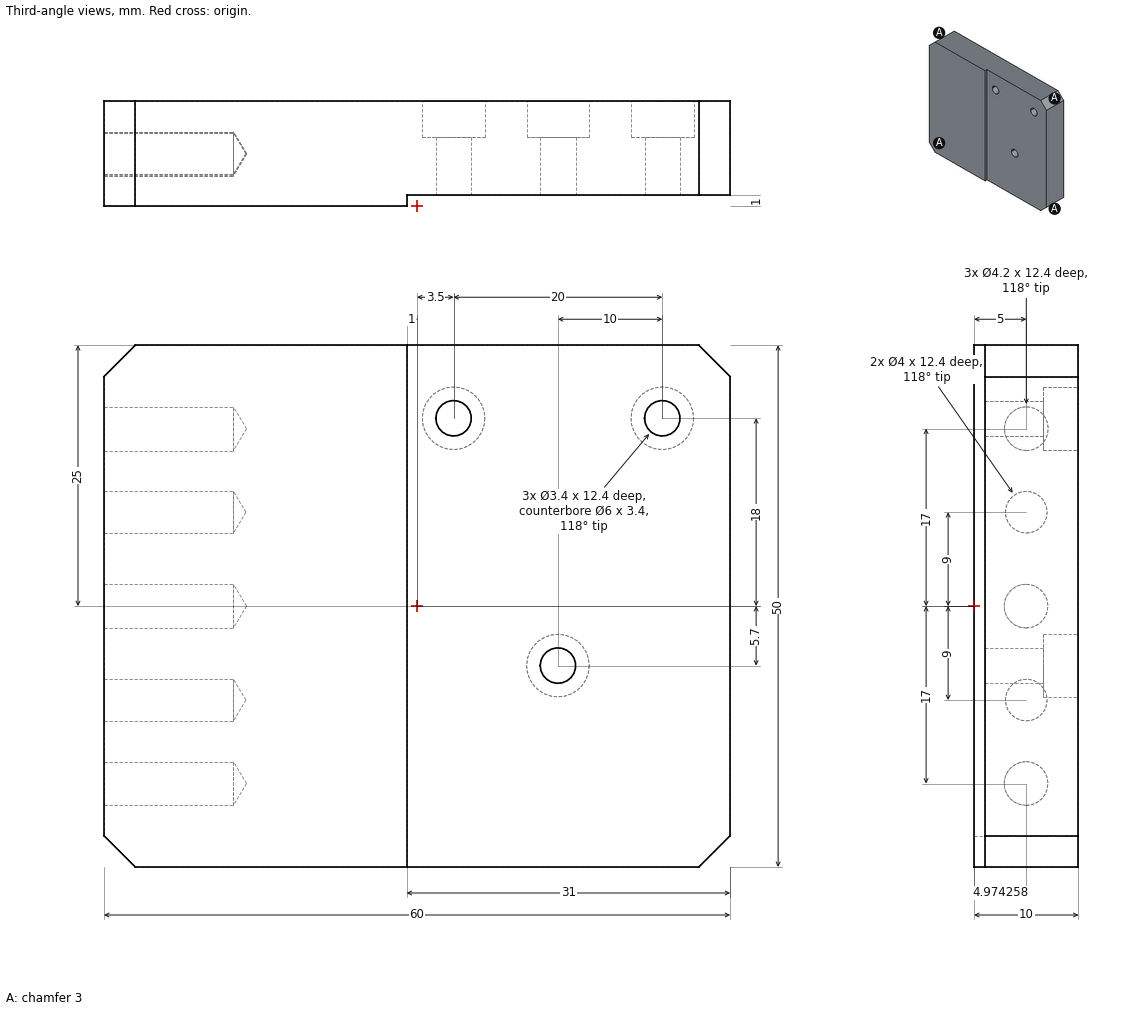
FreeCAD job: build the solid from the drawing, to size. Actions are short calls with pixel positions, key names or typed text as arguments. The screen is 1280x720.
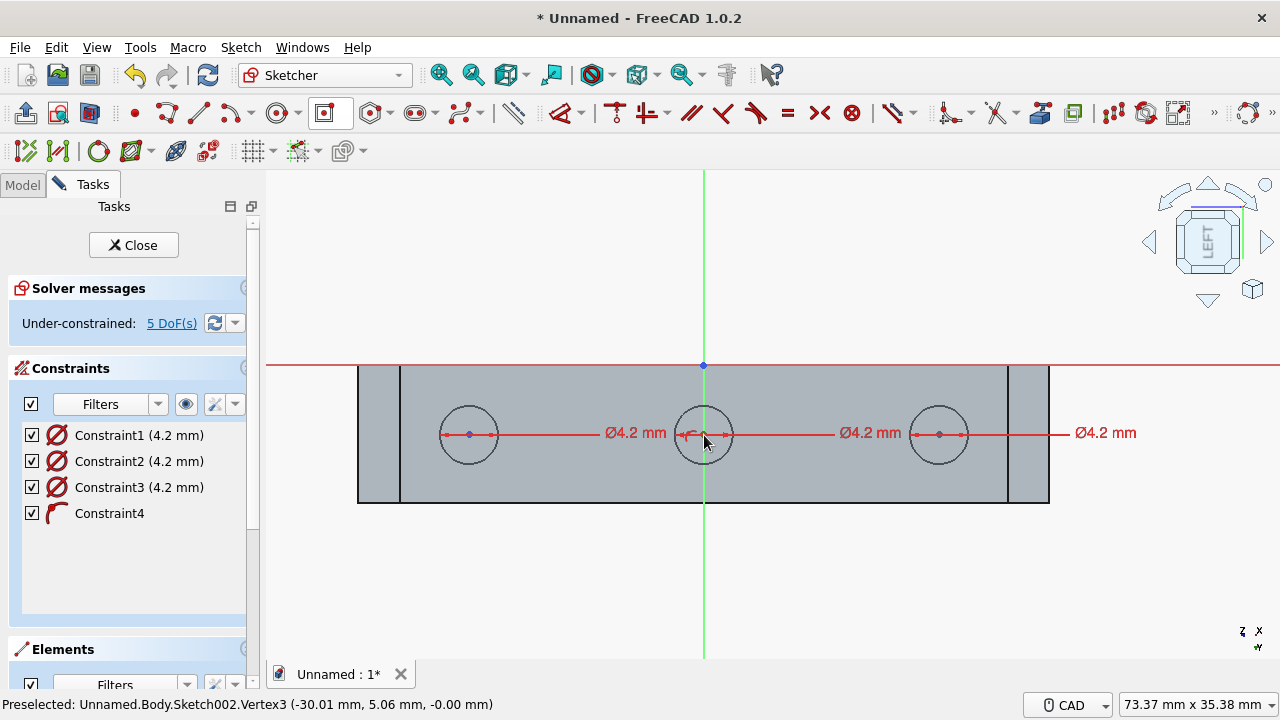
click(670, 114)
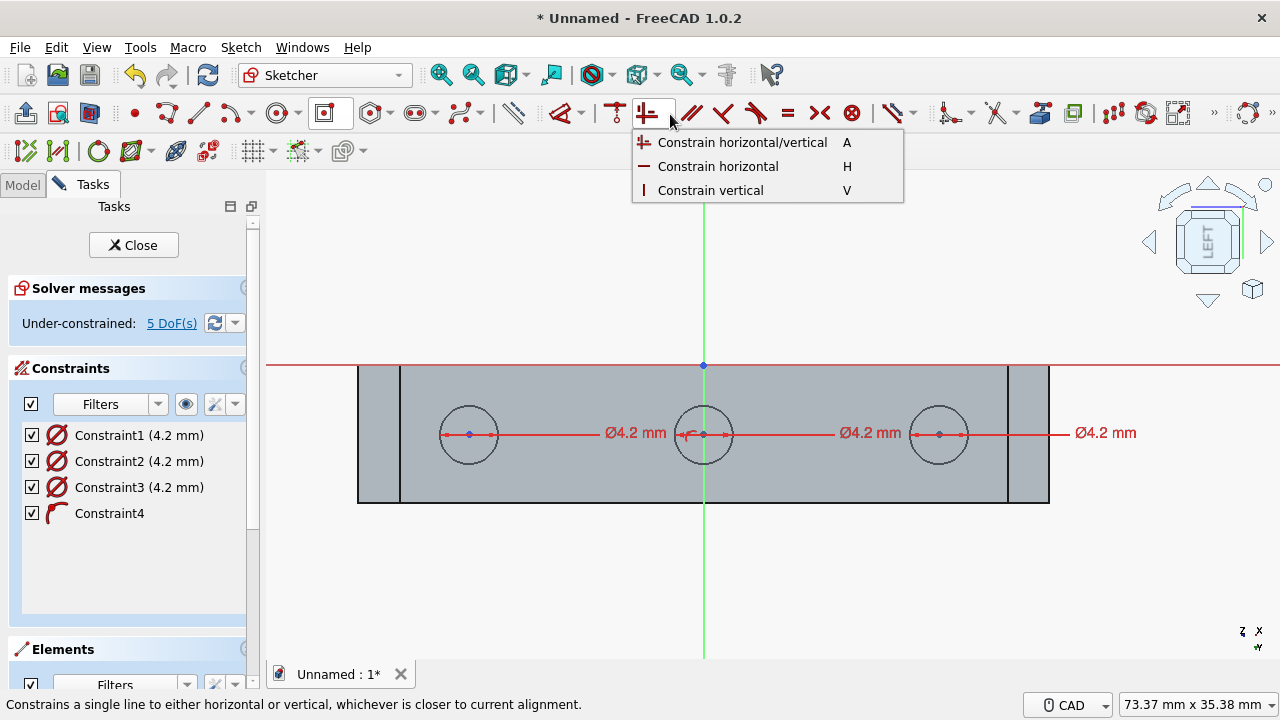
click(768, 166)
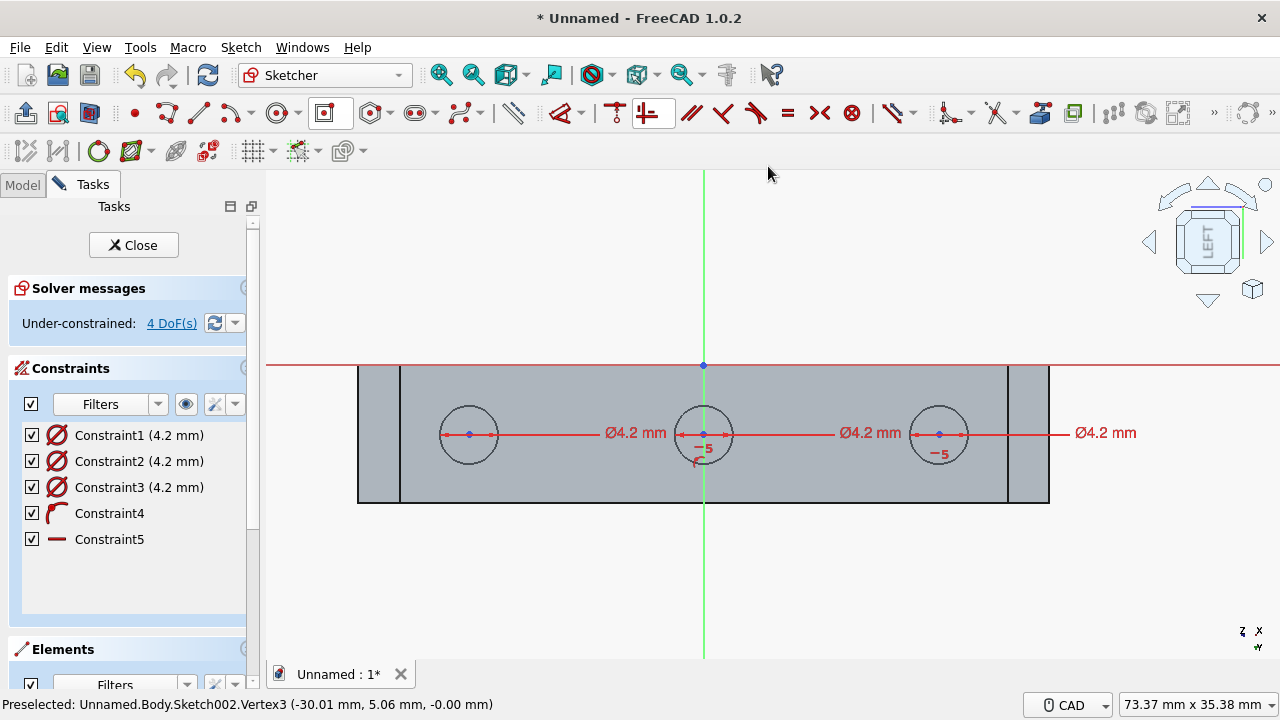
click(560, 114)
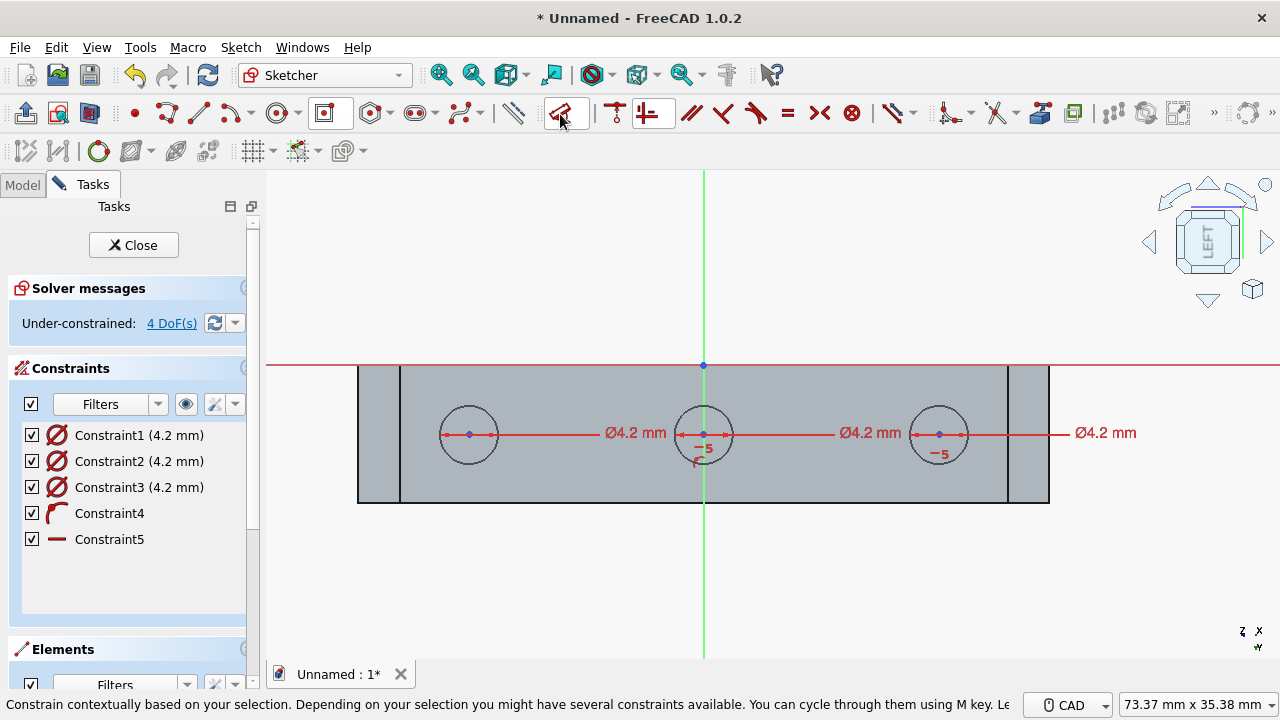
click(469, 435)
click(435, 400)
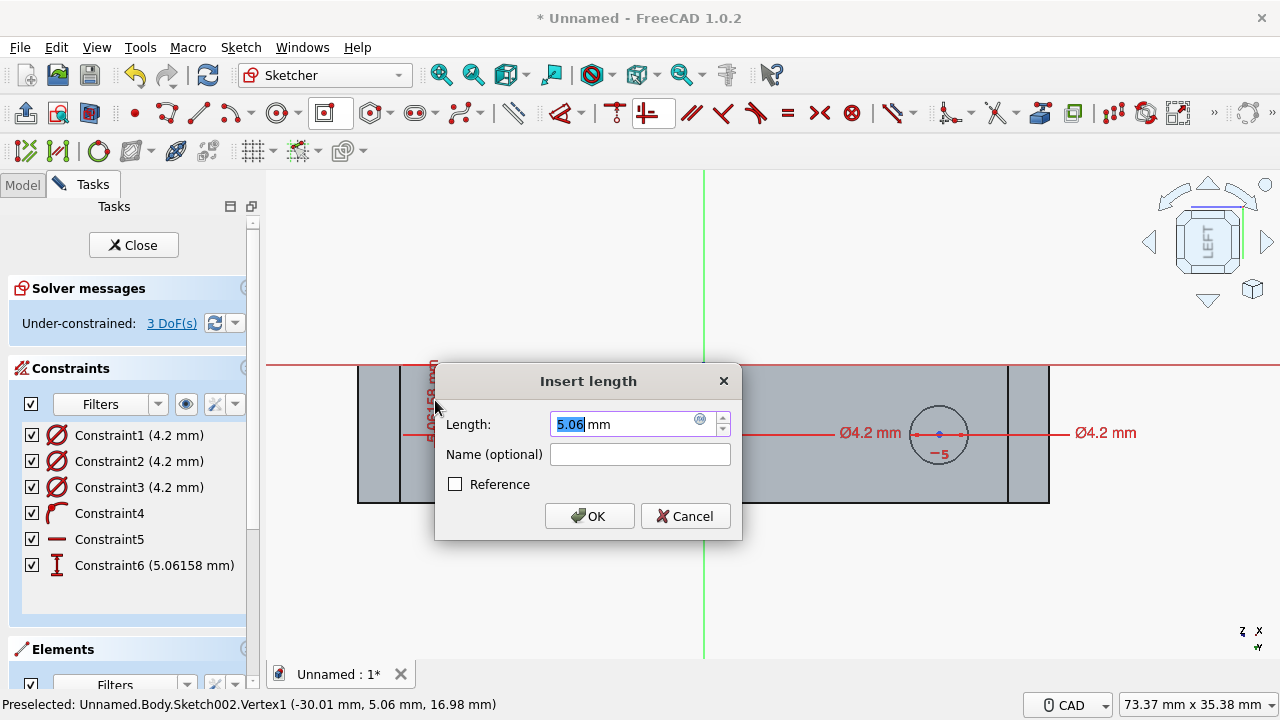
text(5)
key(Return)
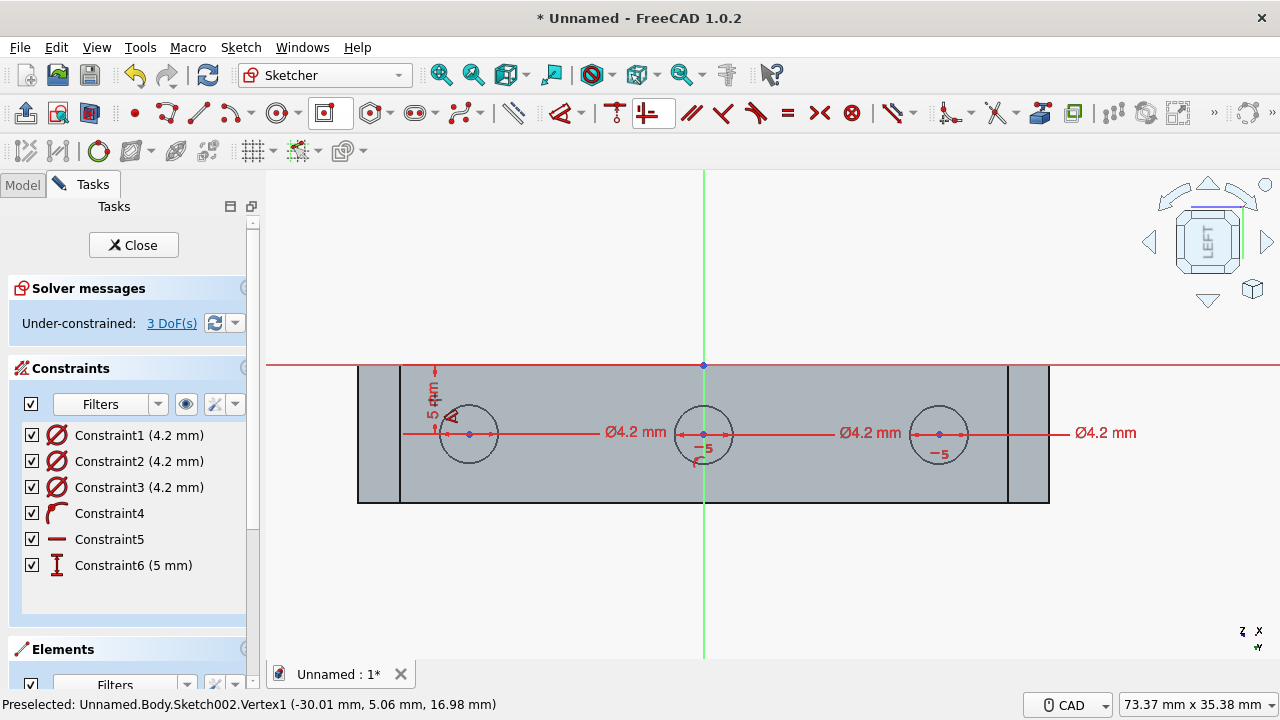
click(469, 434)
click(586, 331)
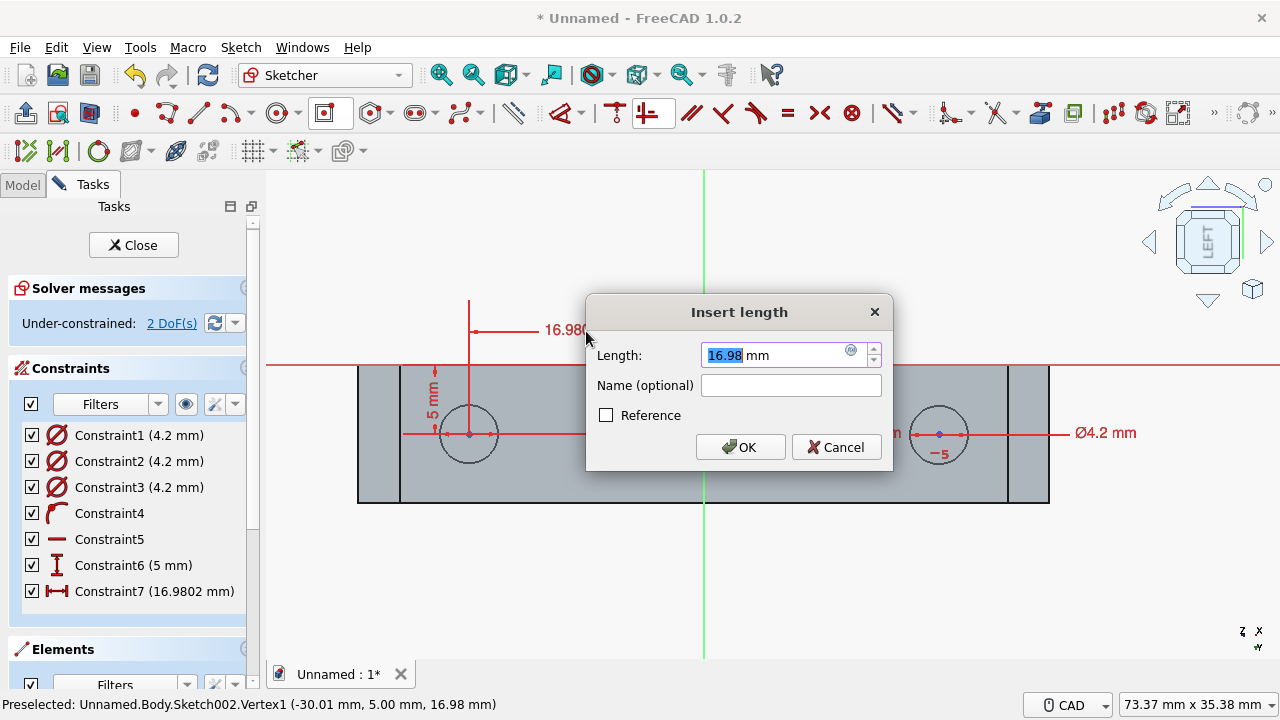
text(17)
key(Return)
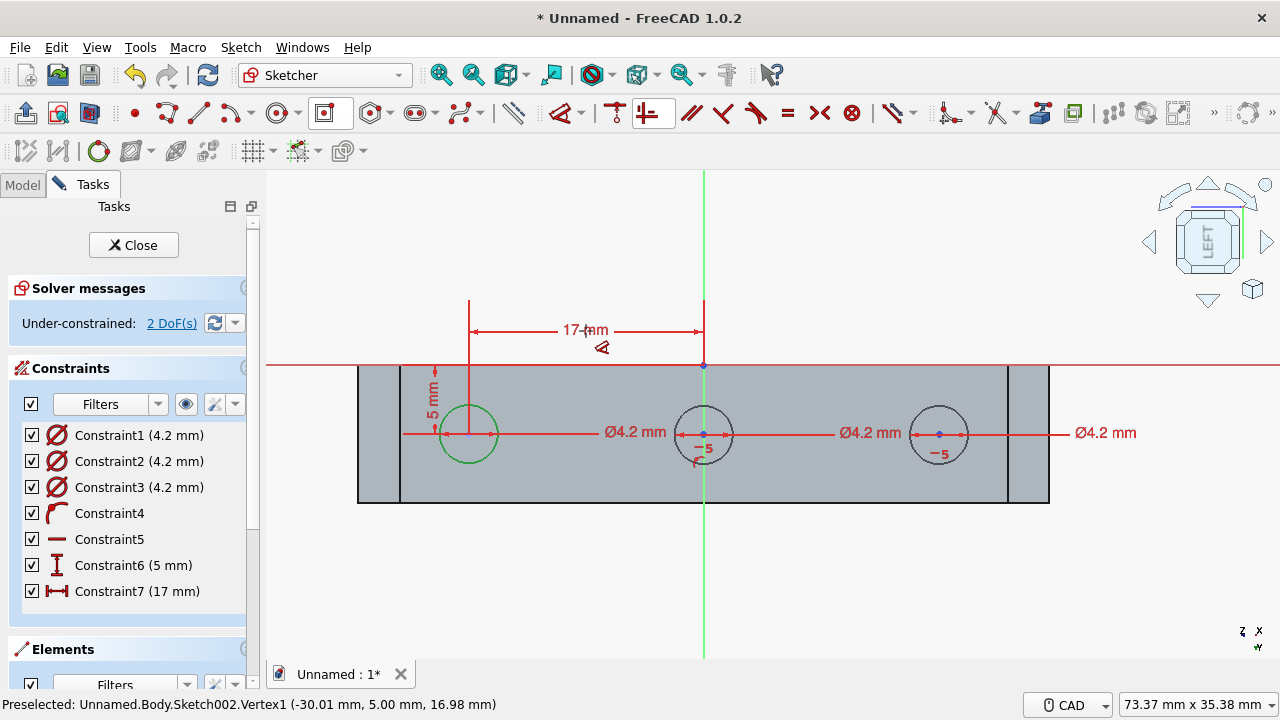
click(939, 435)
click(821, 331)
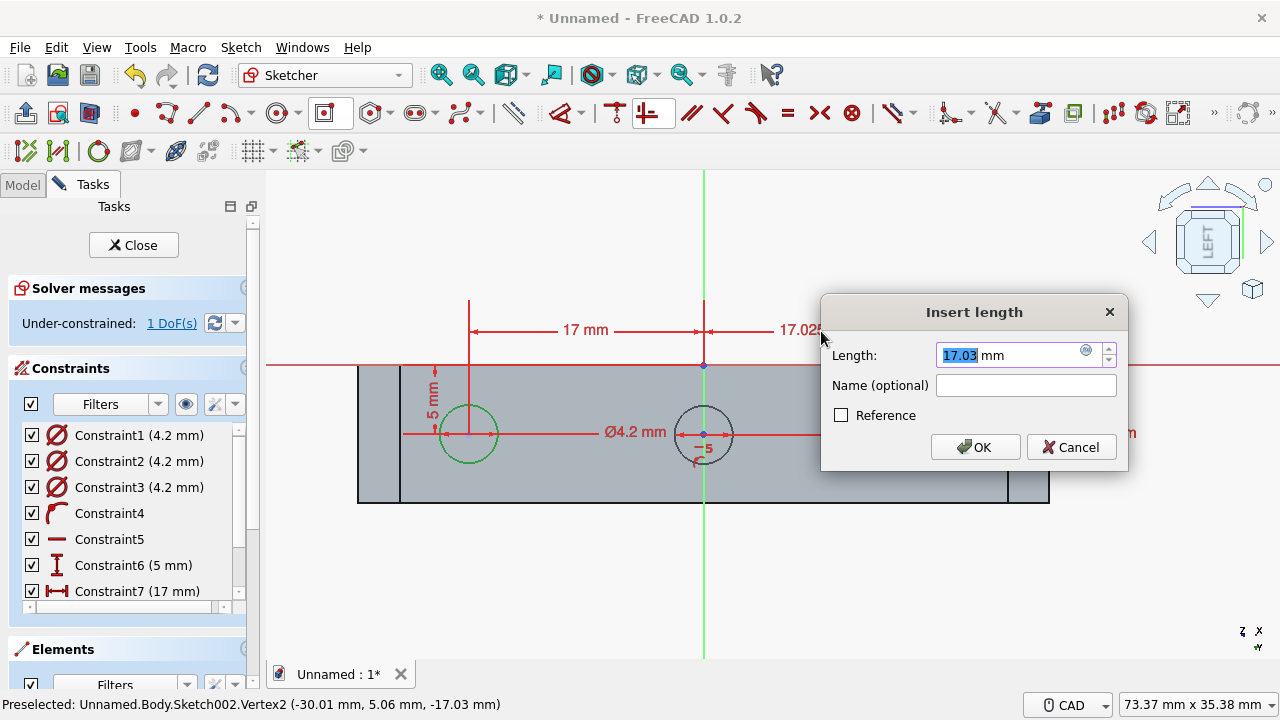
text(17)
key(Return)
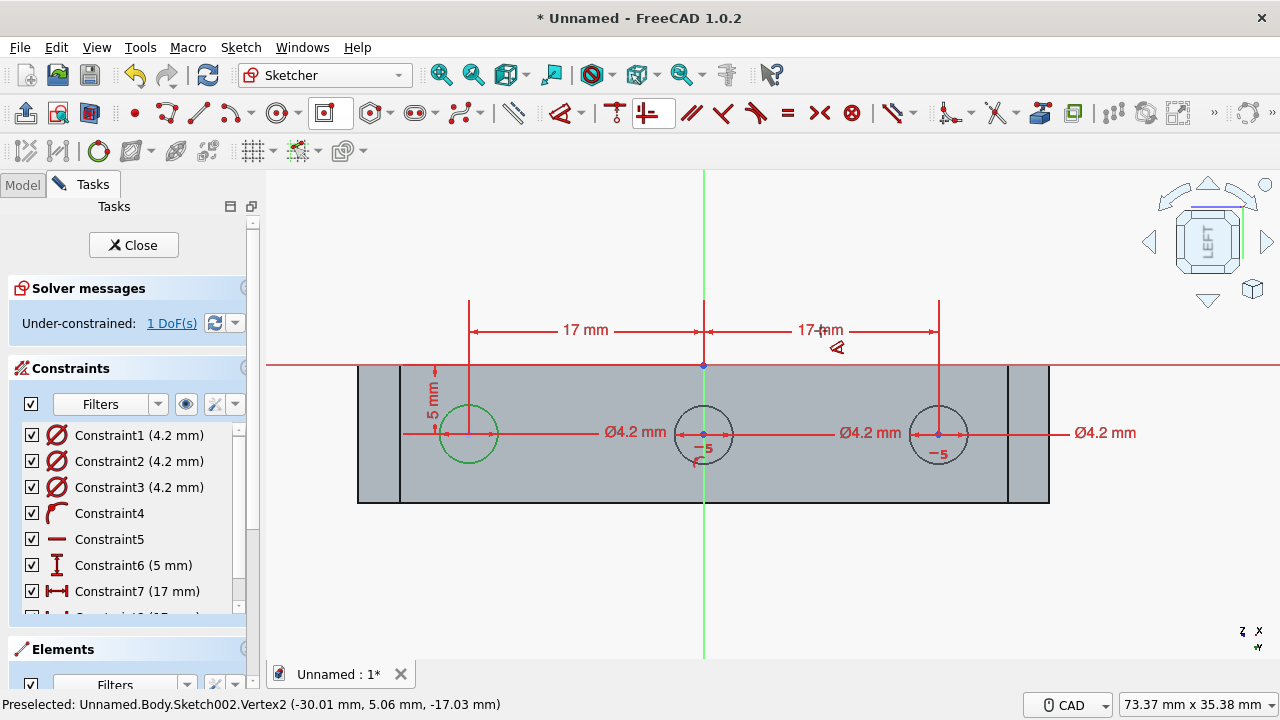
click(939, 435)
click(973, 400)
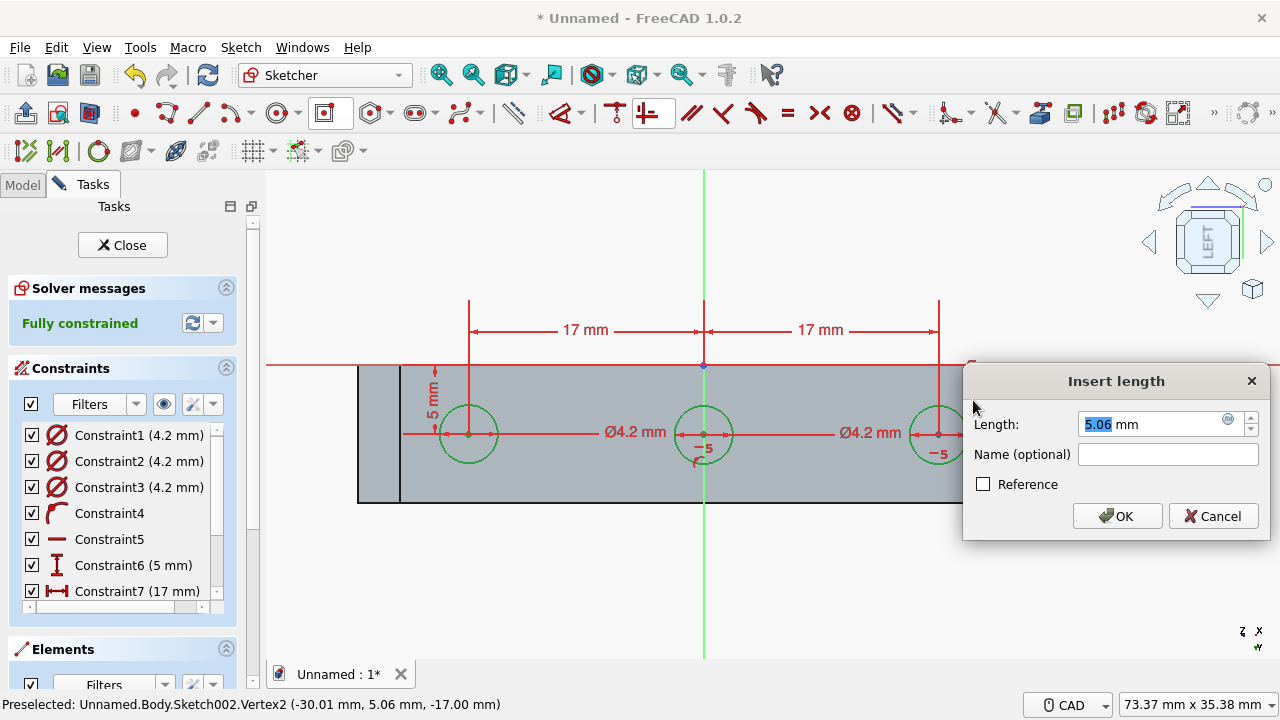
text(4.974258)
key(Return)
key(Escape)